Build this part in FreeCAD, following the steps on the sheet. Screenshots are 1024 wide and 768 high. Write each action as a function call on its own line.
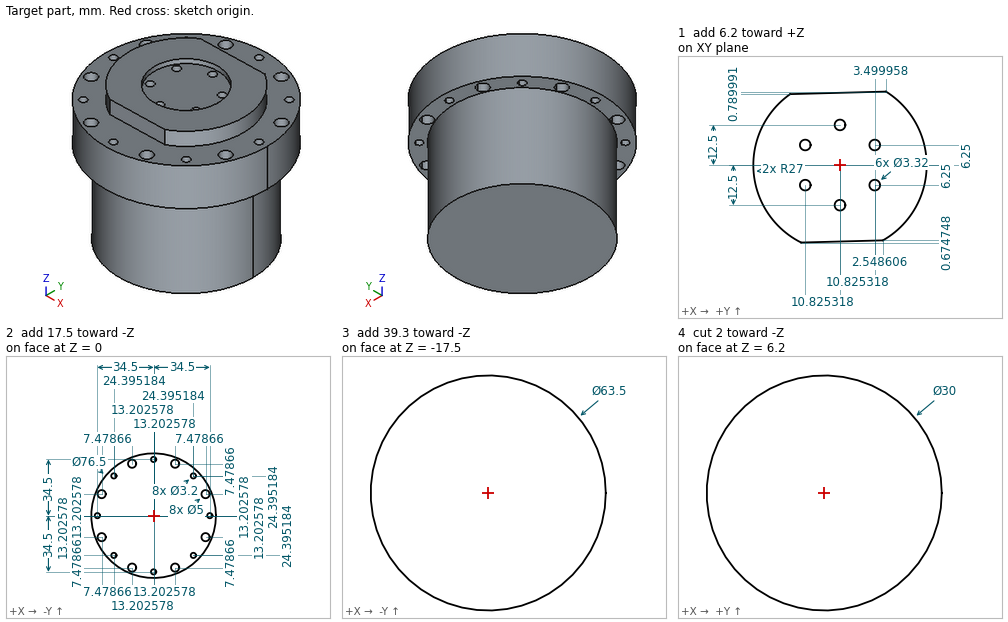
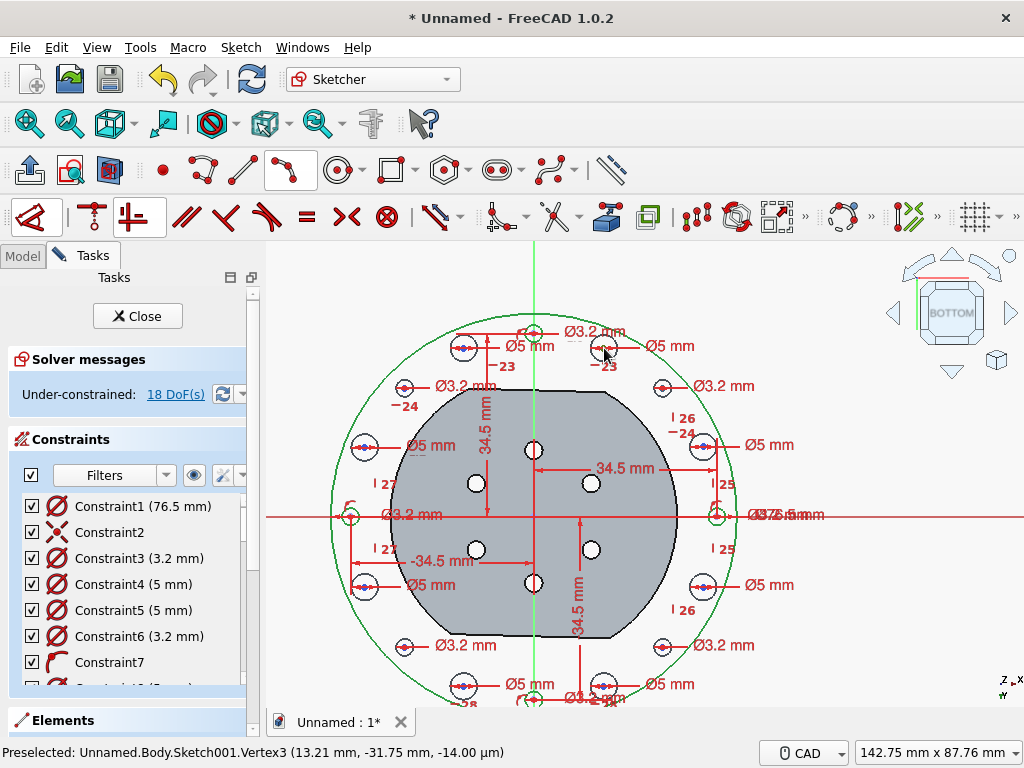
key(i)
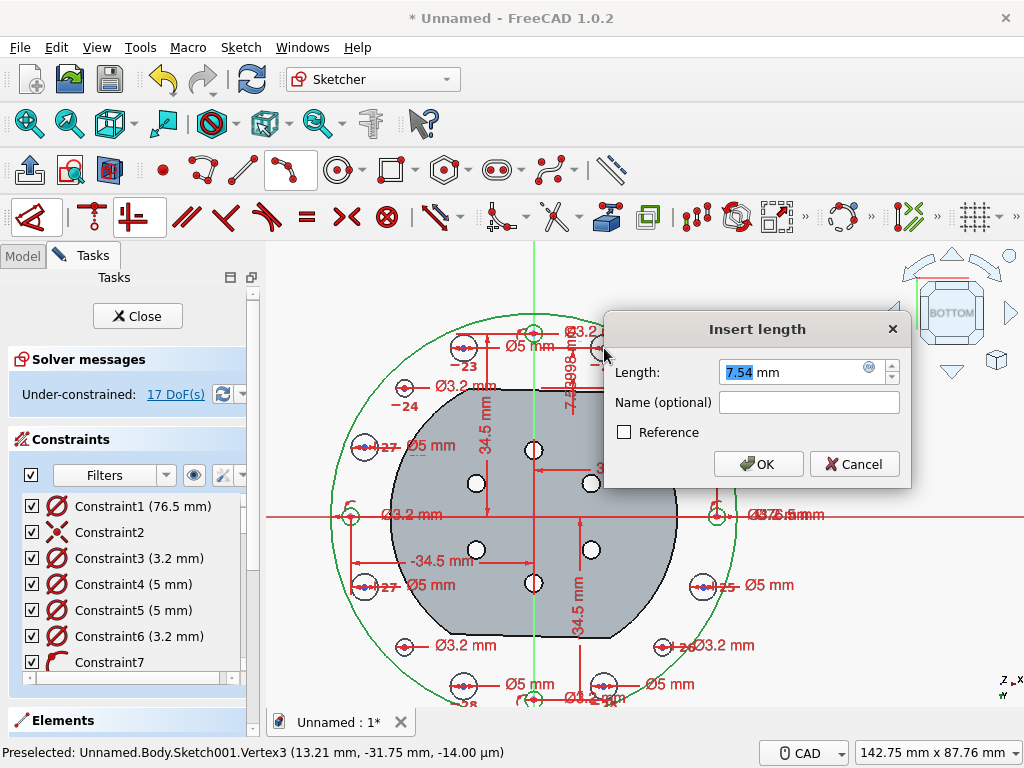
text(7.47866)
key(Return)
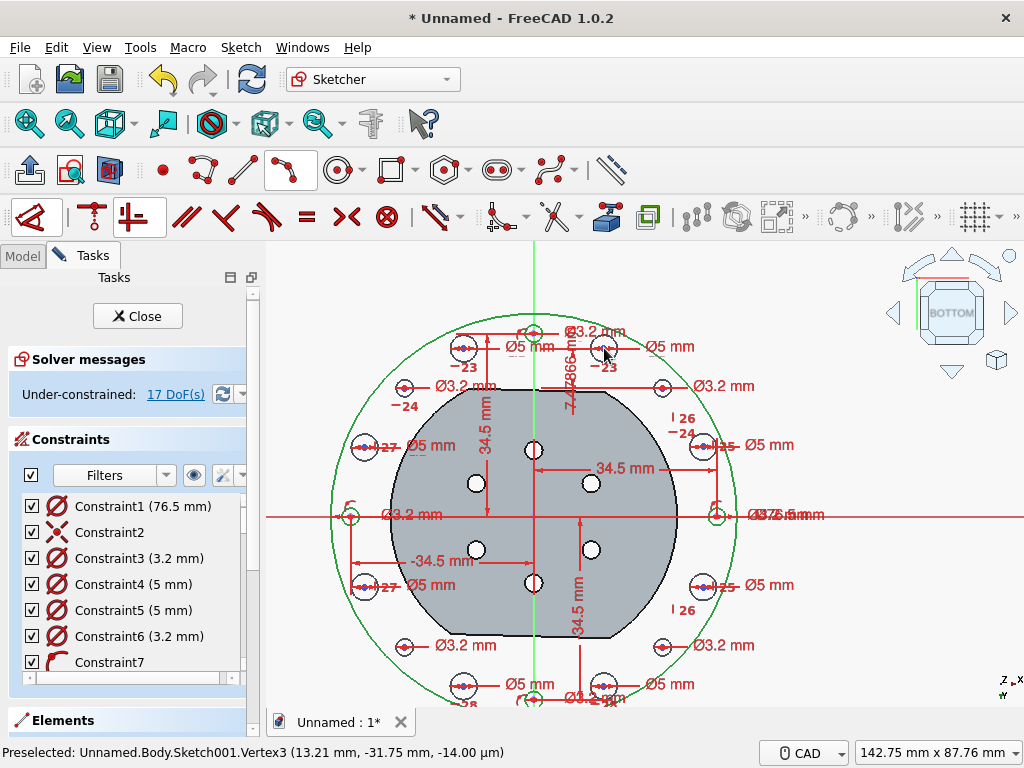
click(663, 388)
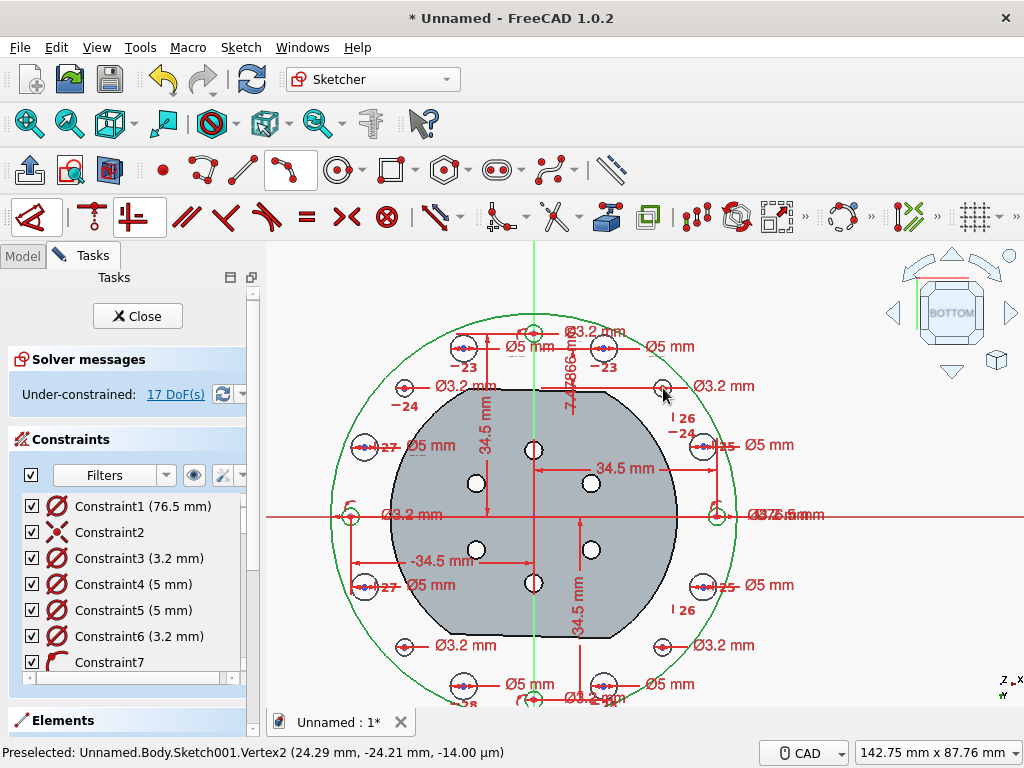
click(703, 447)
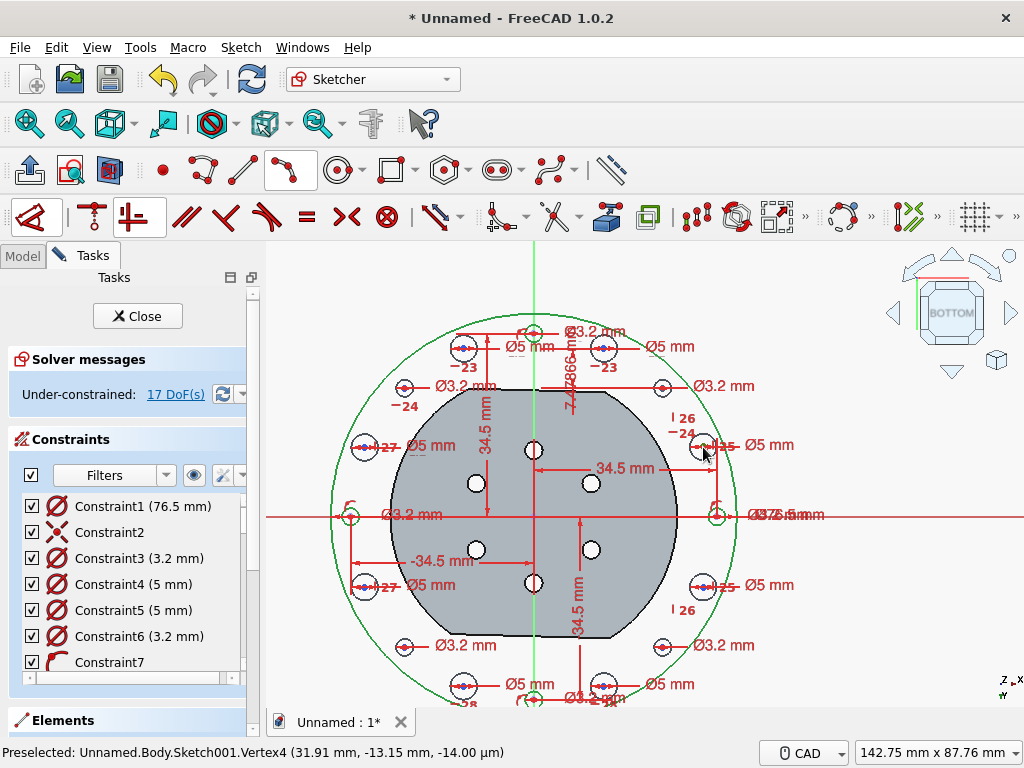
click(56, 218)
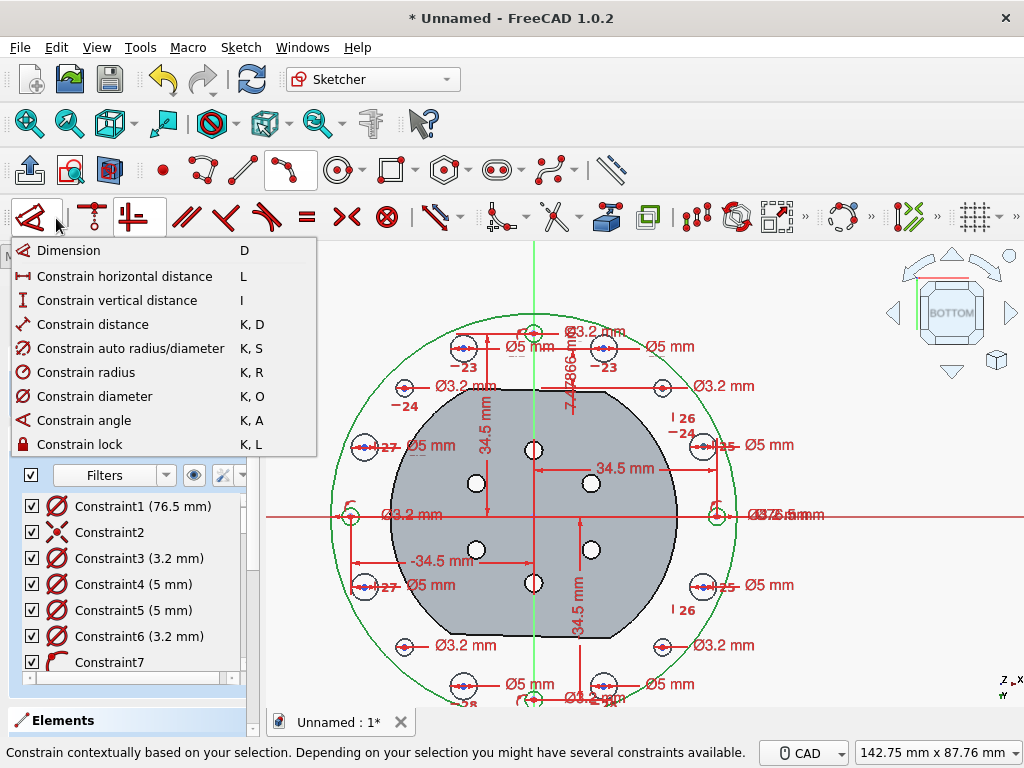
click(164, 276)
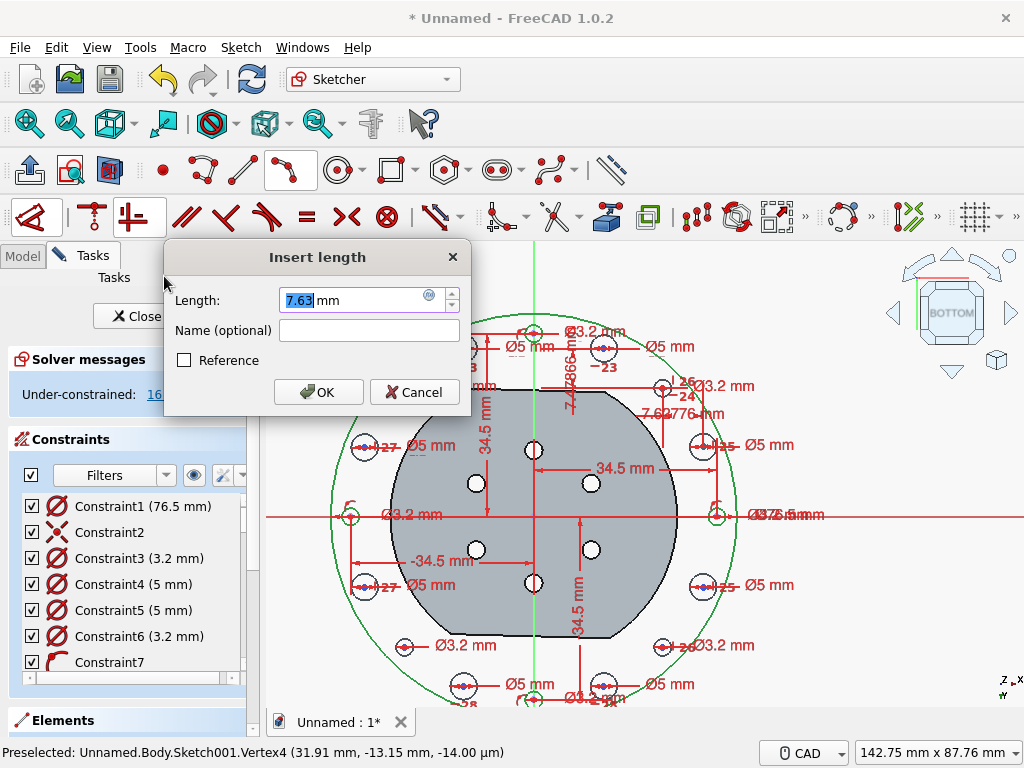
text(7.47866)
key(Return)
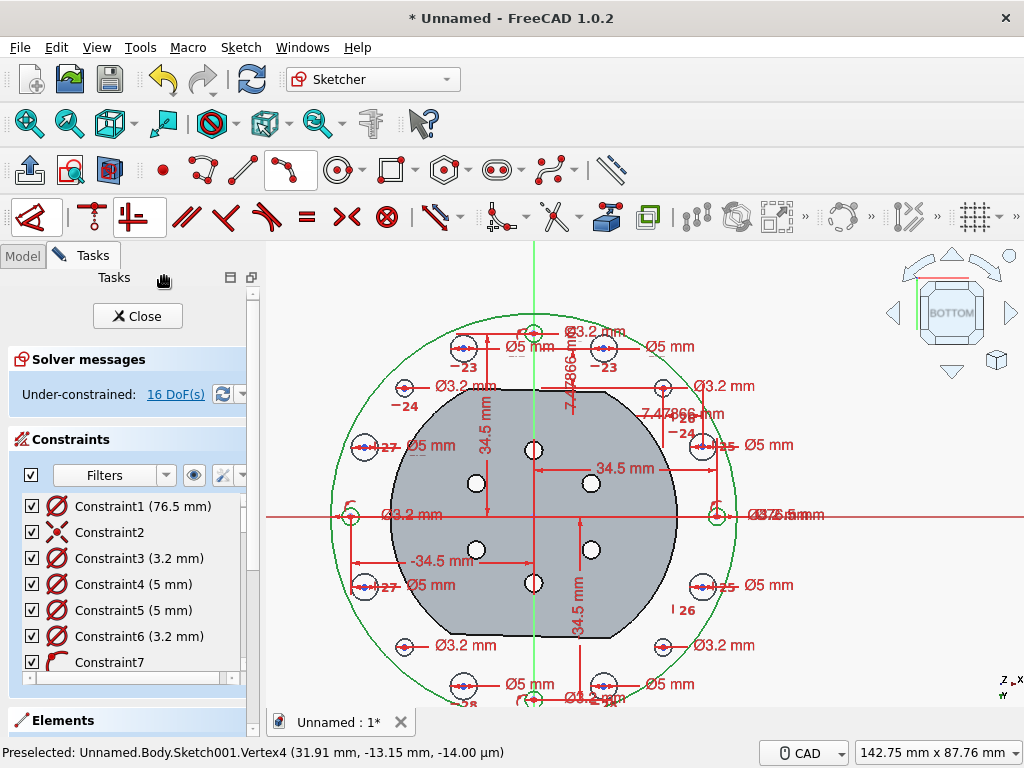
click(405, 388)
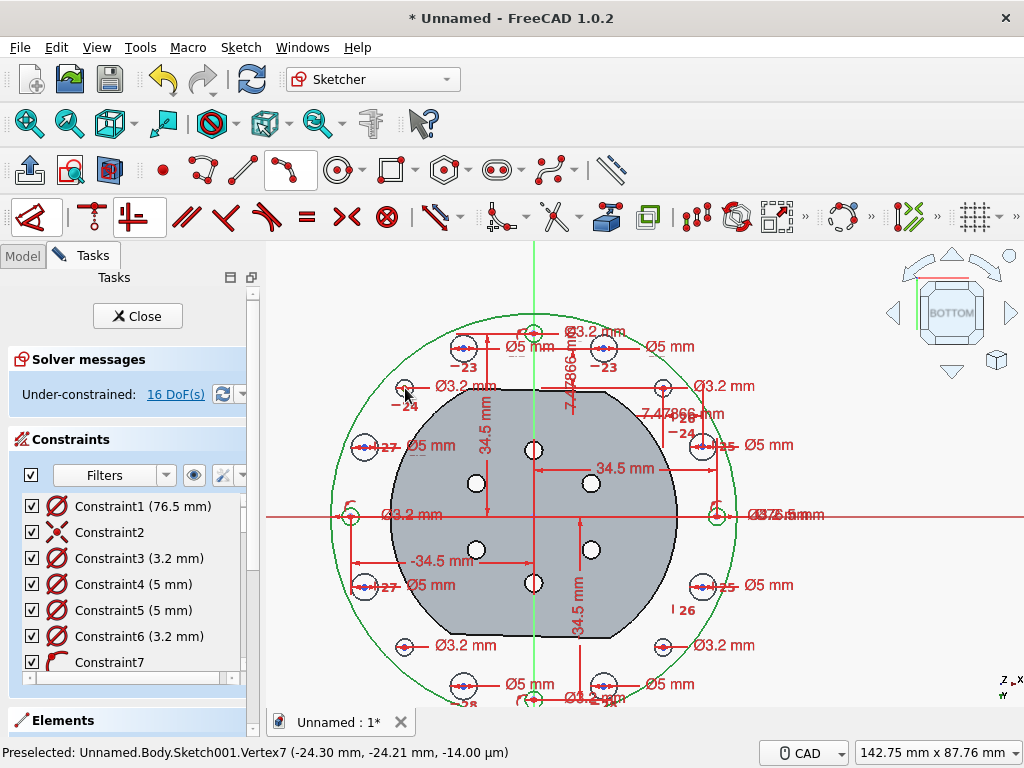
click(365, 448)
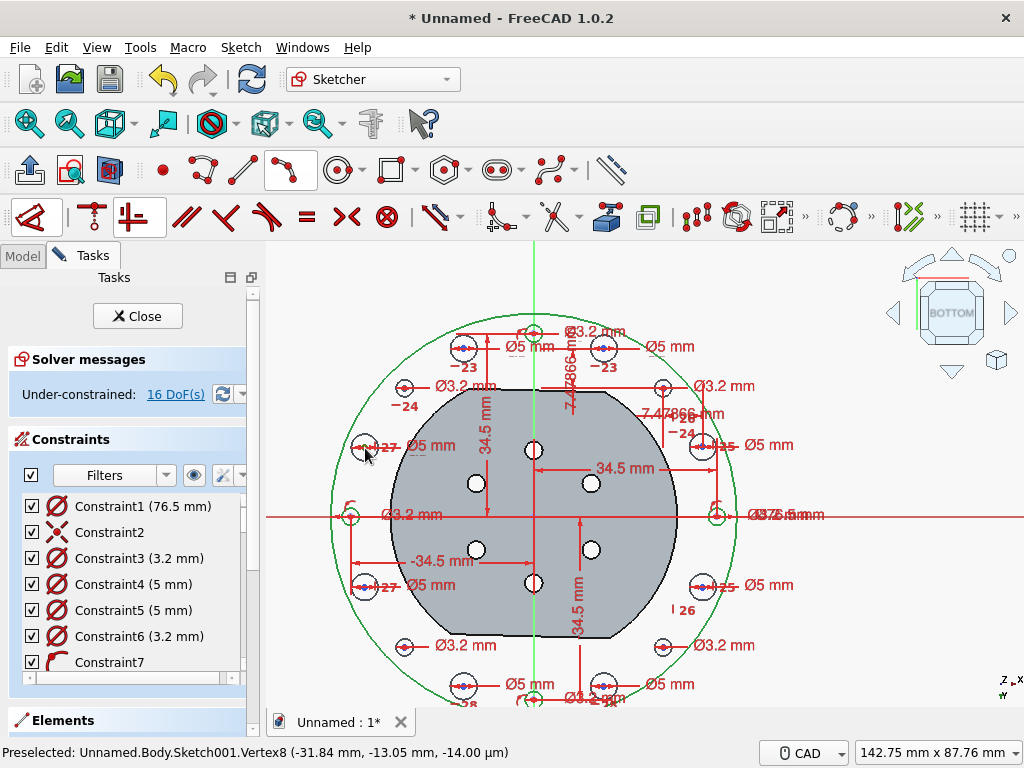
key(l)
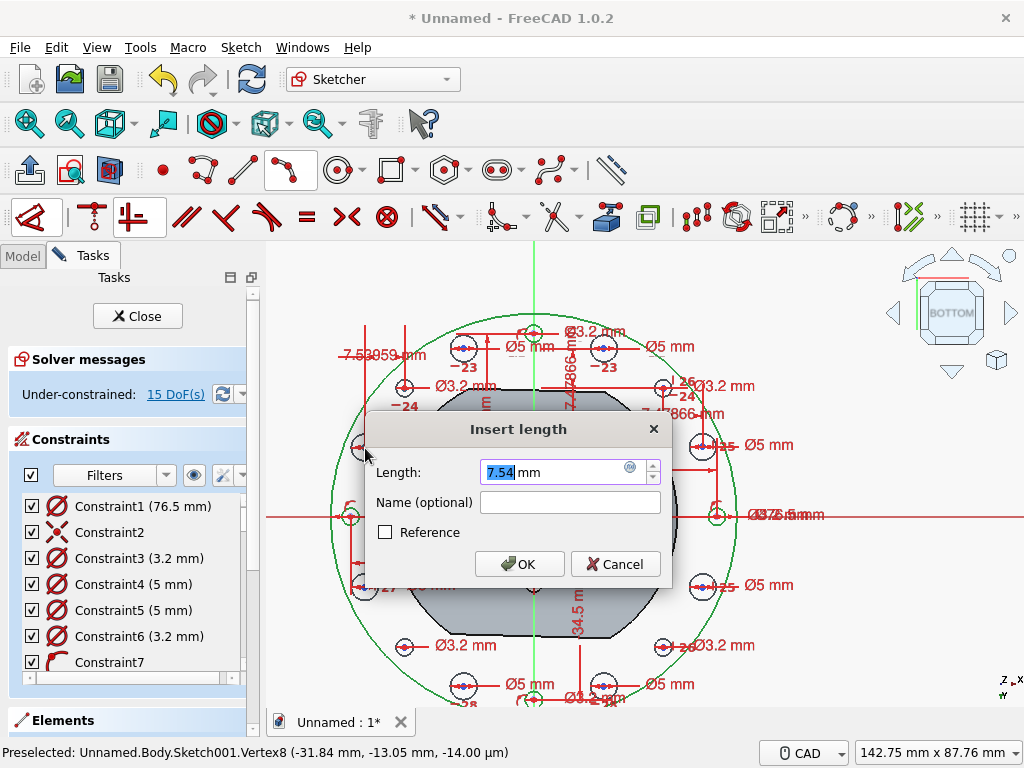
text(7.47866)
key(Return)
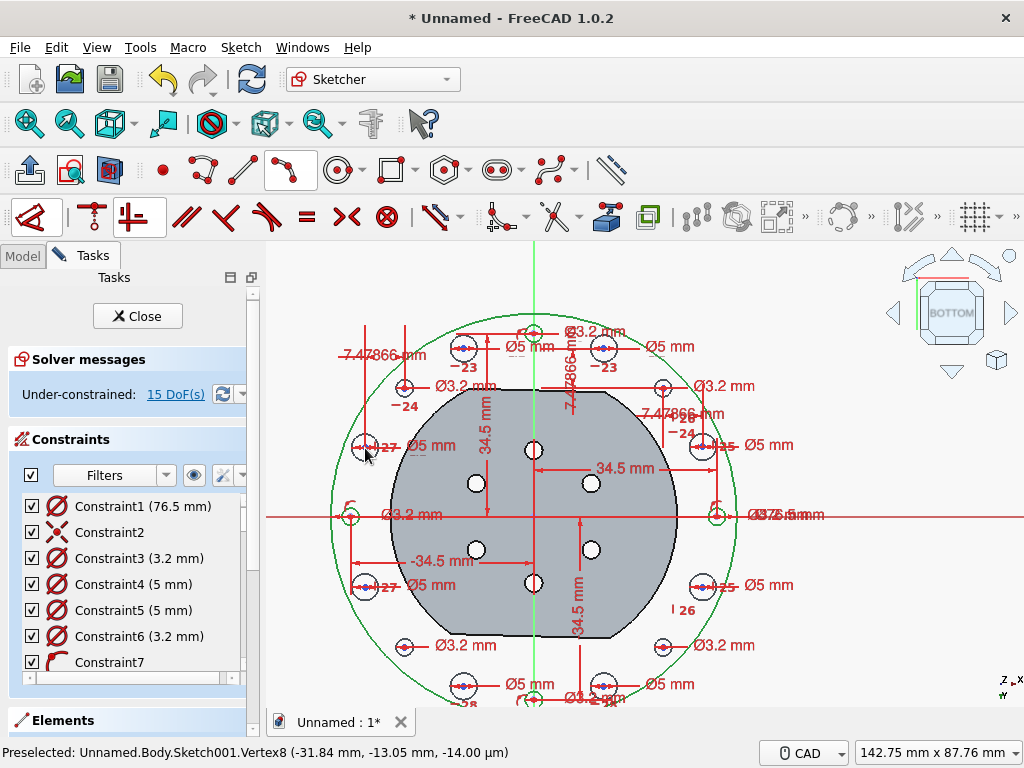
click(663, 647)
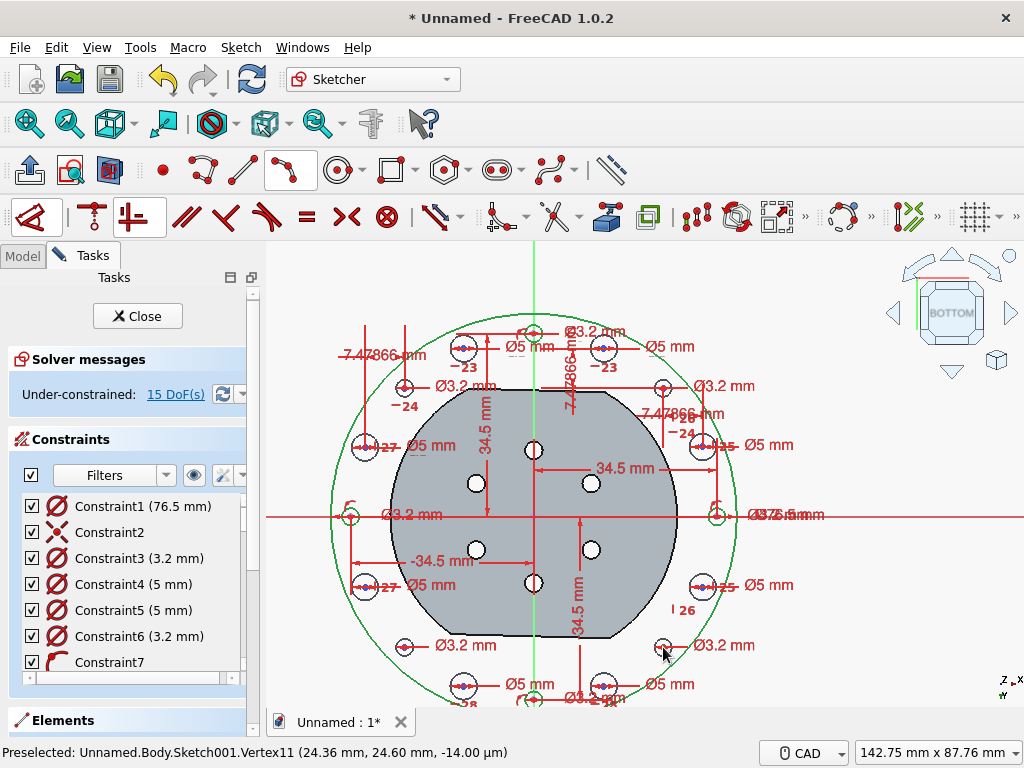
scroll(663, 387, down, 2)